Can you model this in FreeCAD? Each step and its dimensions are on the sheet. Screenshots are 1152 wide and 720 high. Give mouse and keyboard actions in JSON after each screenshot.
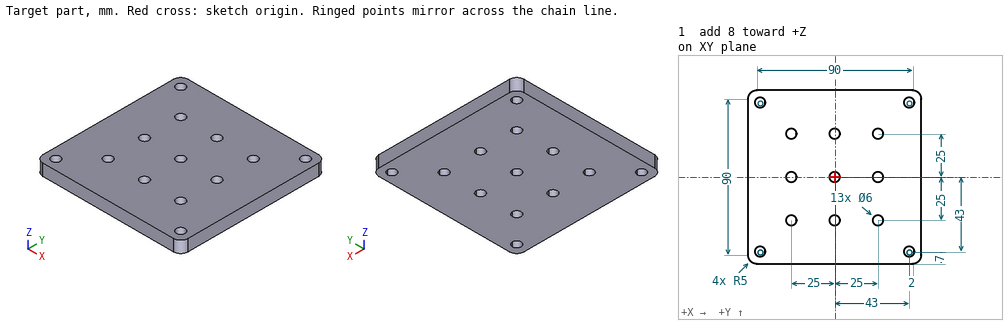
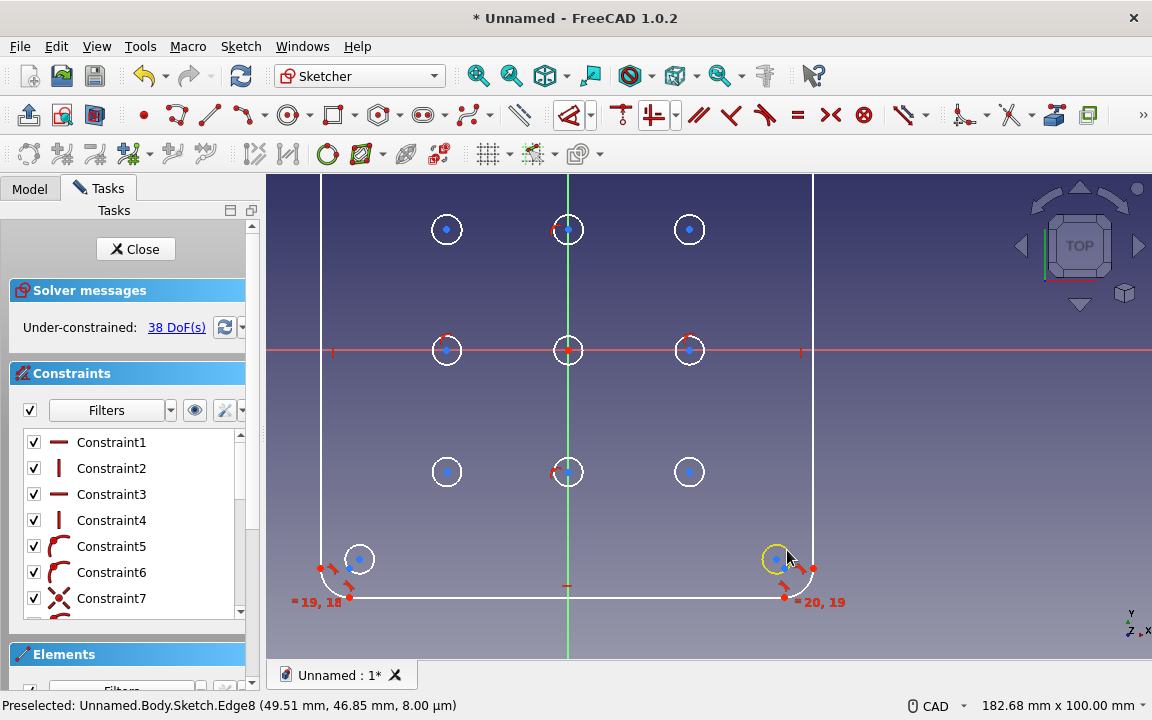
{"action": "left_click", "coordinate": [787, 549]}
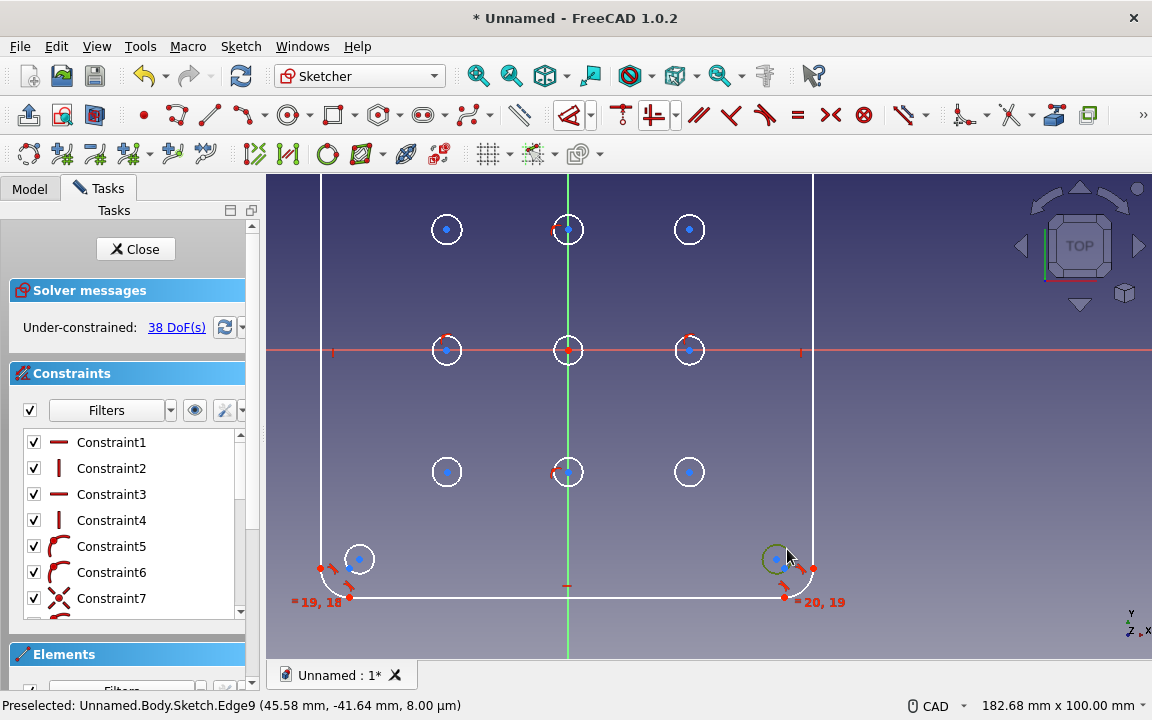
{"action": "left_click", "coordinate": [700, 462]}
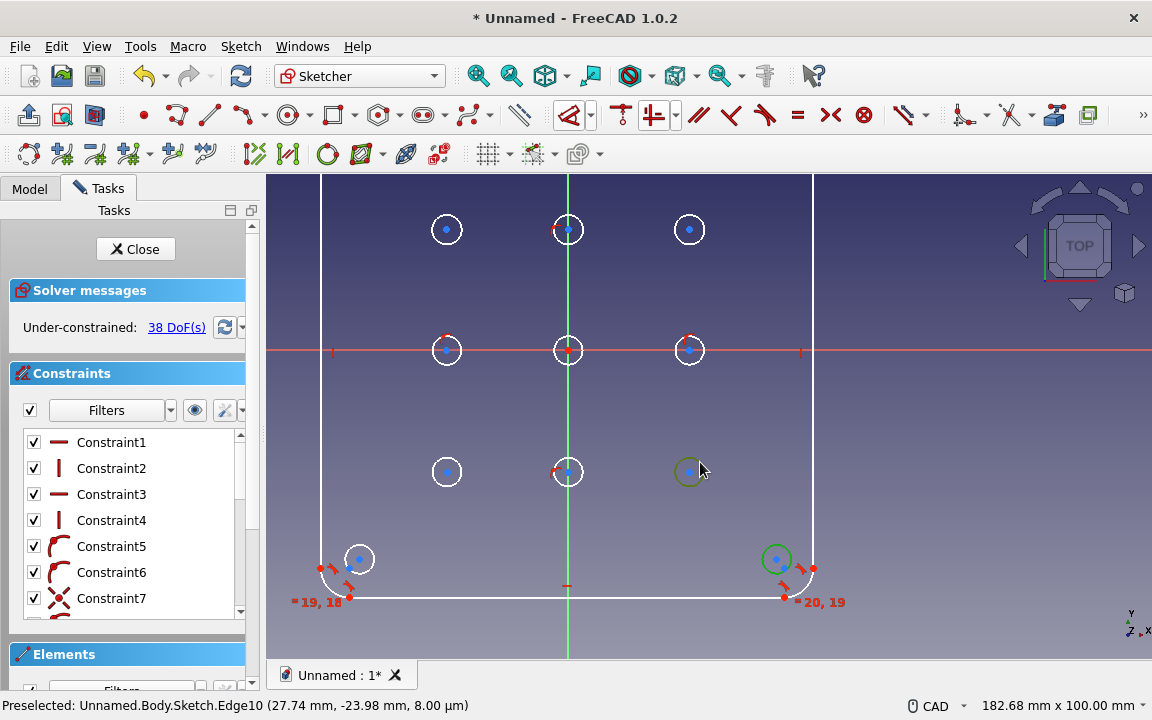
{"action": "scroll", "coordinate": [578, 462], "scroll_direction": "up", "scroll_amount": 2}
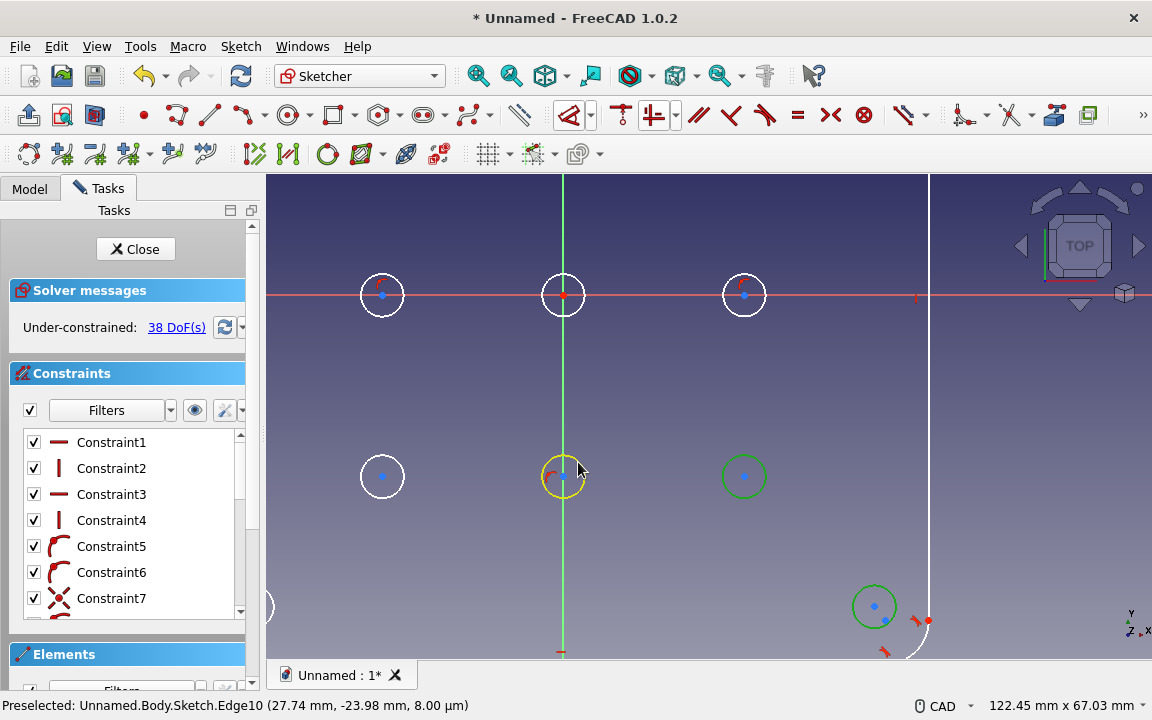
{"action": "left_click", "coordinate": [578, 462]}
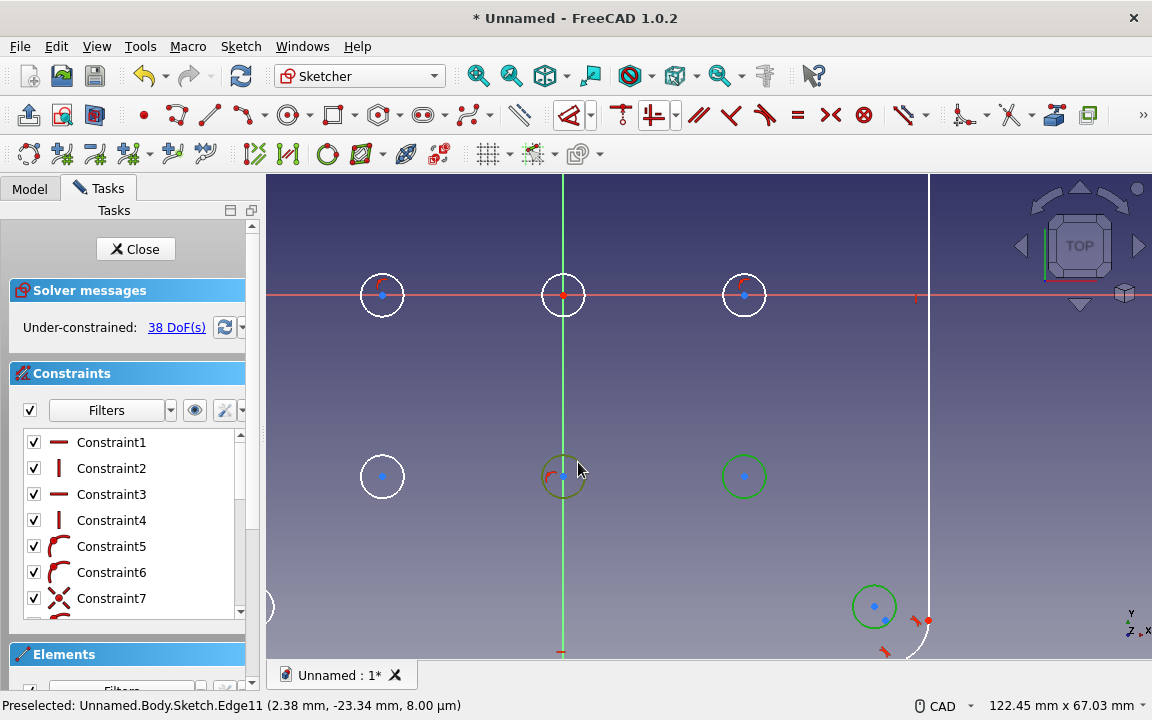
{"action": "scroll", "coordinate": [703, 515], "scroll_direction": "down", "scroll_amount": 4}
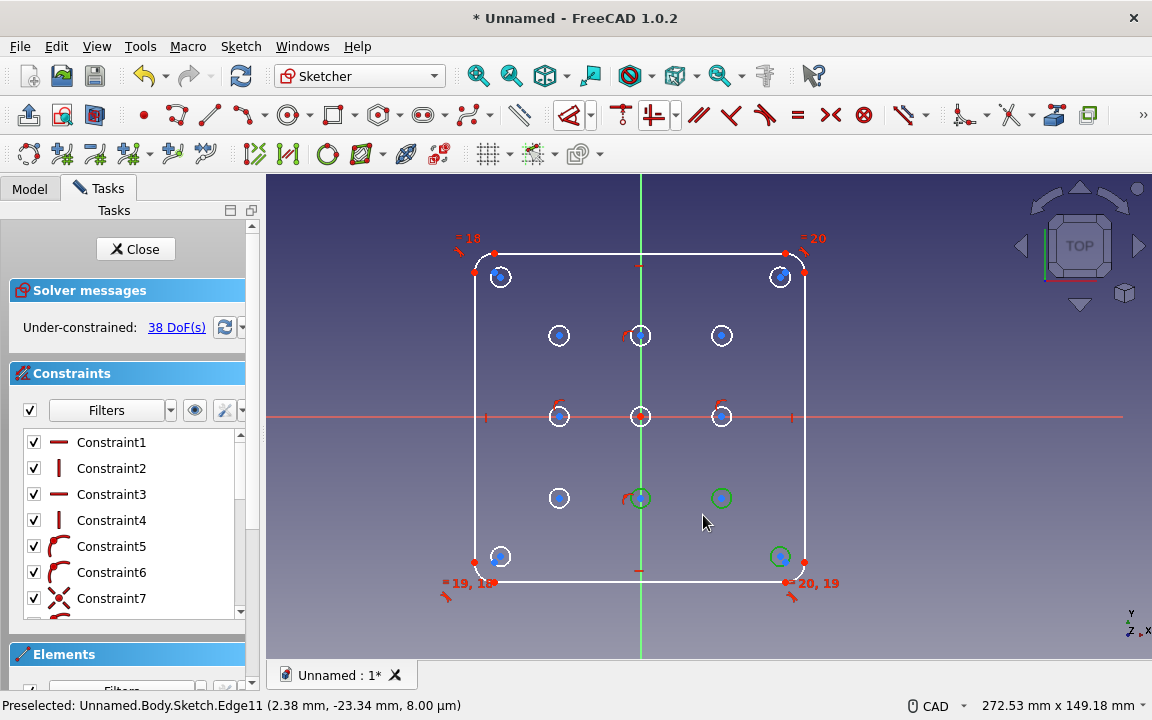
{"action": "scroll", "coordinate": [508, 550], "scroll_direction": "up", "scroll_amount": 2}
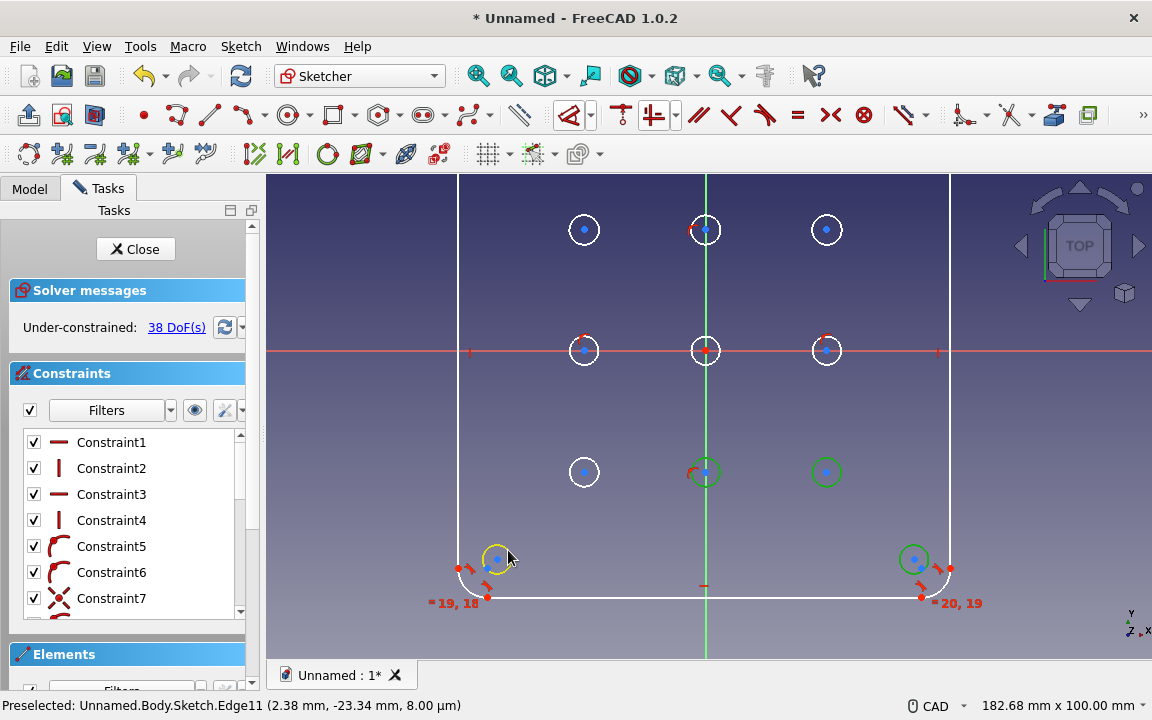
{"action": "left_click", "coordinate": [507, 549]}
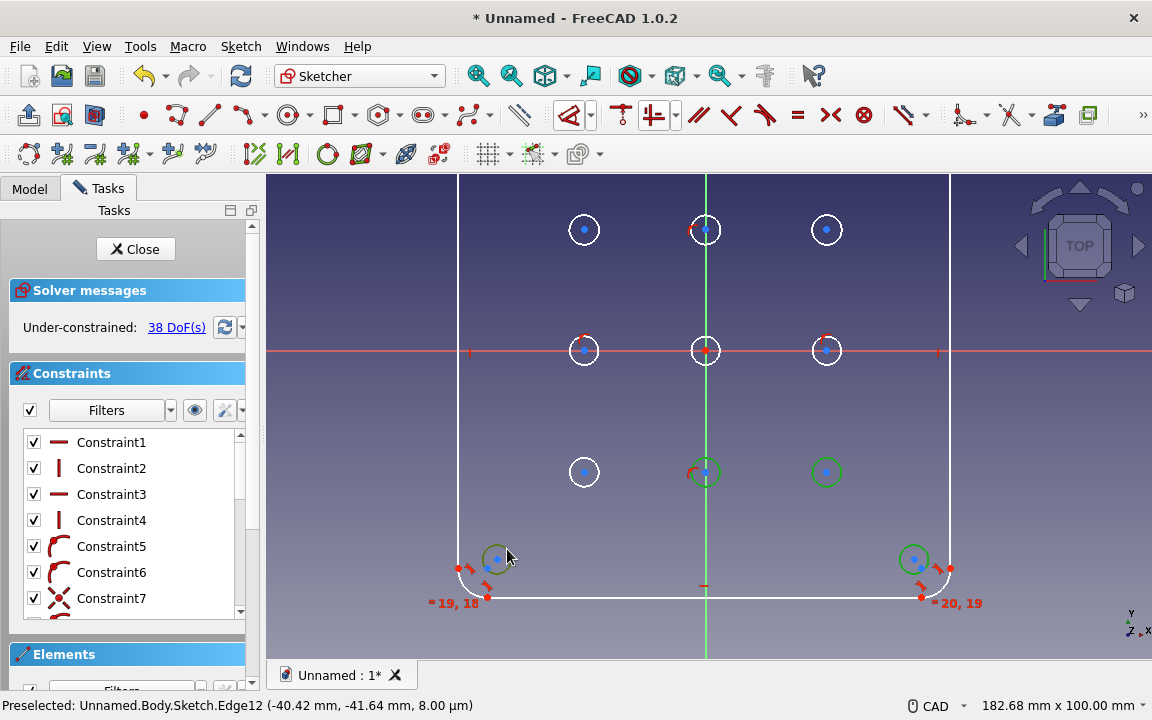
{"action": "left_click", "coordinate": [594, 462]}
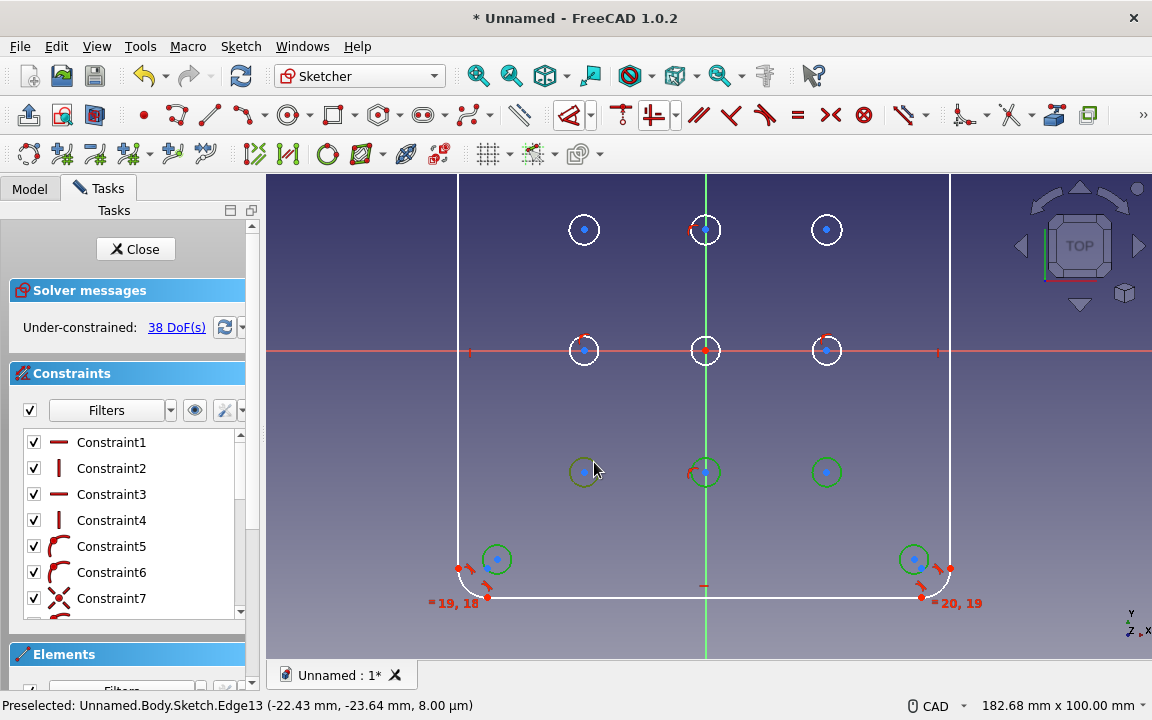
{"action": "scroll", "coordinate": [837, 341], "scroll_direction": "up", "scroll_amount": 2}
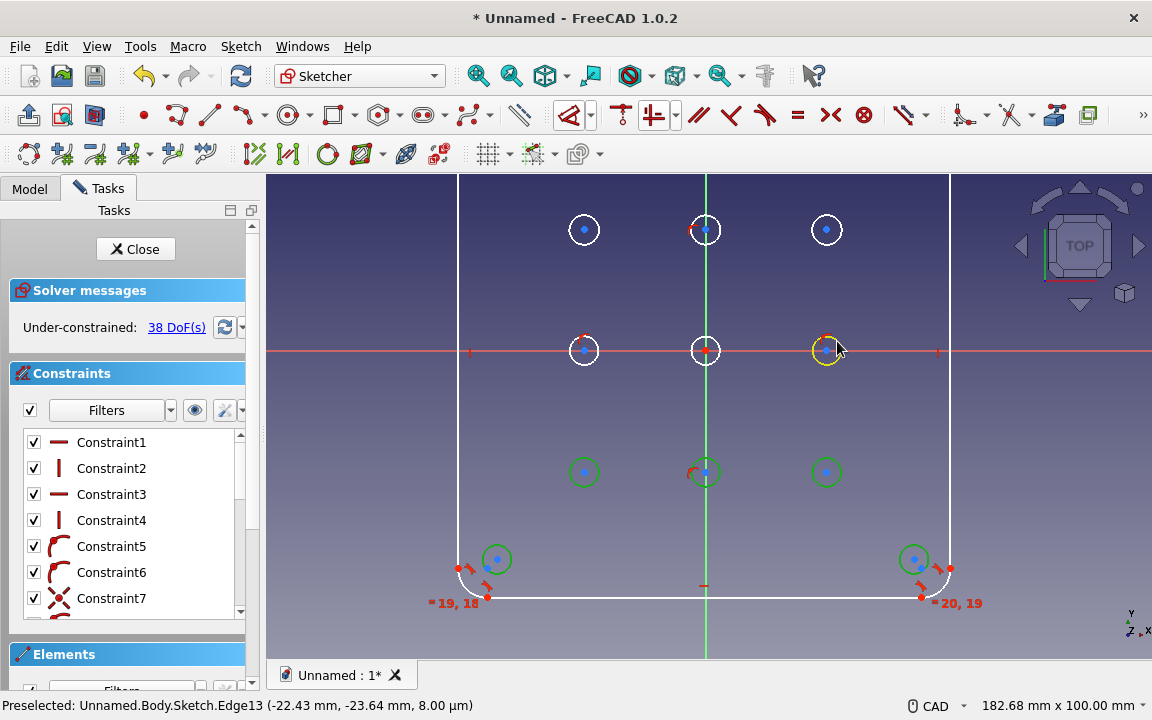
{"action": "left_click", "coordinate": [837, 340]}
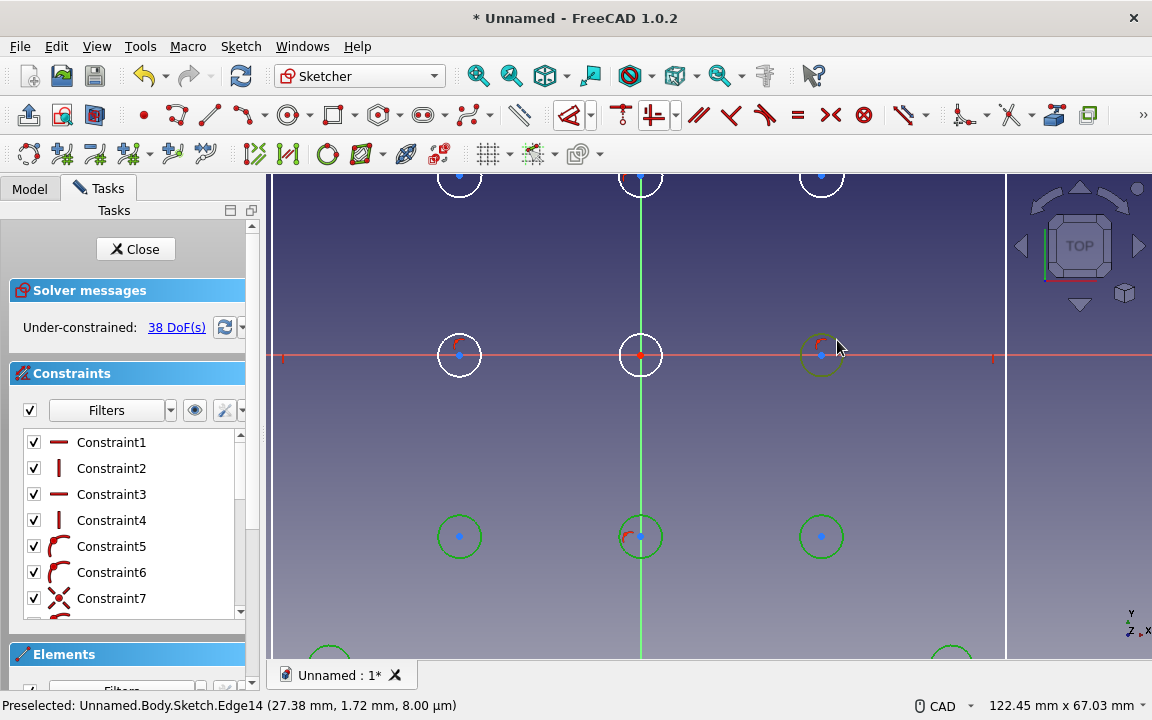
{"action": "scroll", "coordinate": [640, 466], "scroll_direction": "down", "scroll_amount": 4}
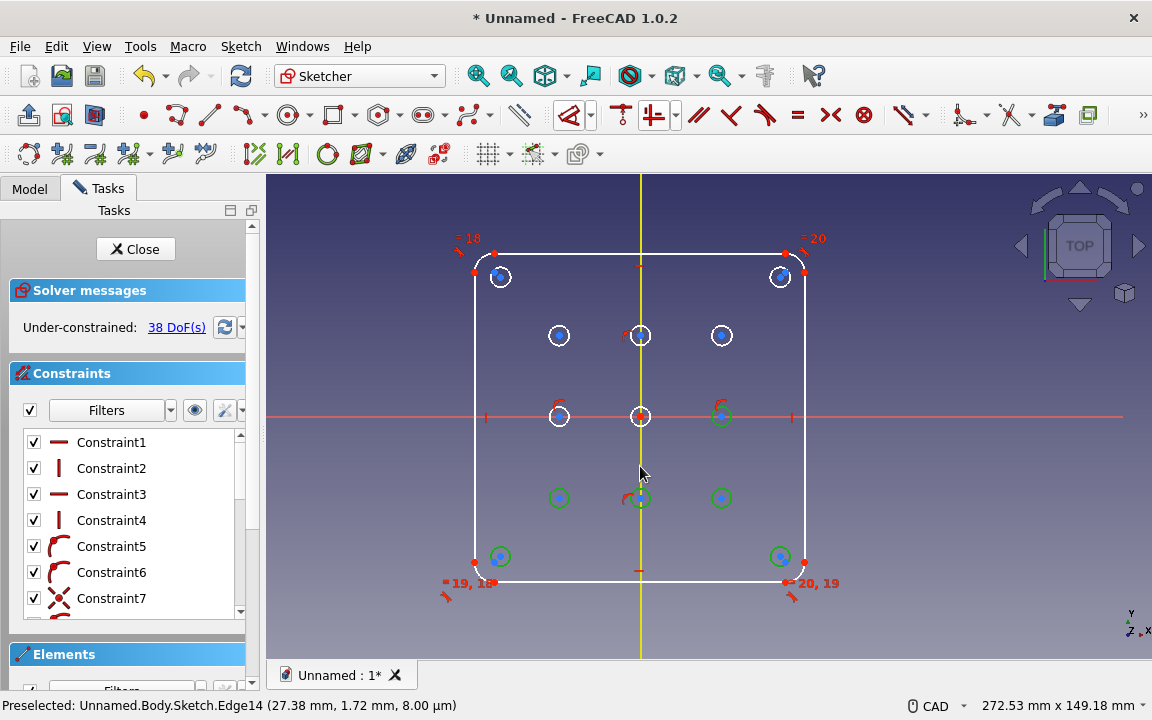
{"action": "scroll", "coordinate": [729, 329], "scroll_direction": "up", "scroll_amount": 2}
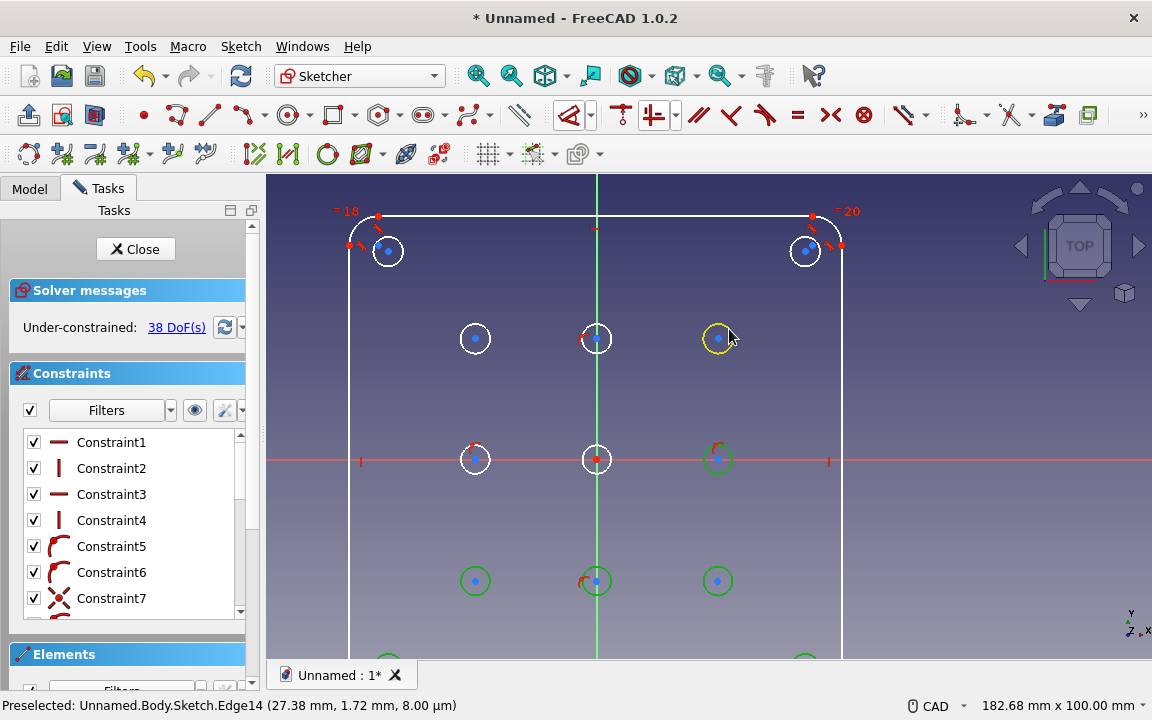
{"action": "left_click", "coordinate": [729, 328]}